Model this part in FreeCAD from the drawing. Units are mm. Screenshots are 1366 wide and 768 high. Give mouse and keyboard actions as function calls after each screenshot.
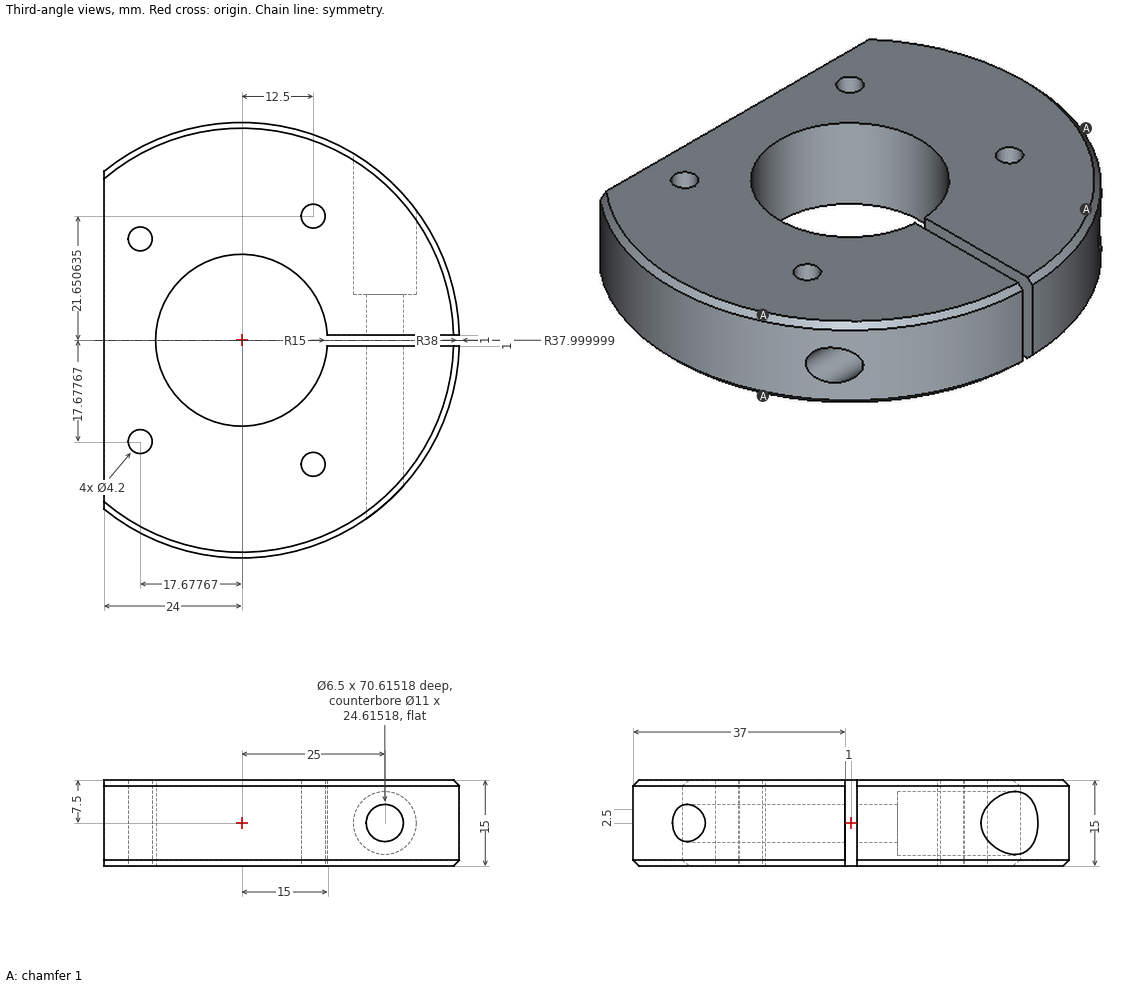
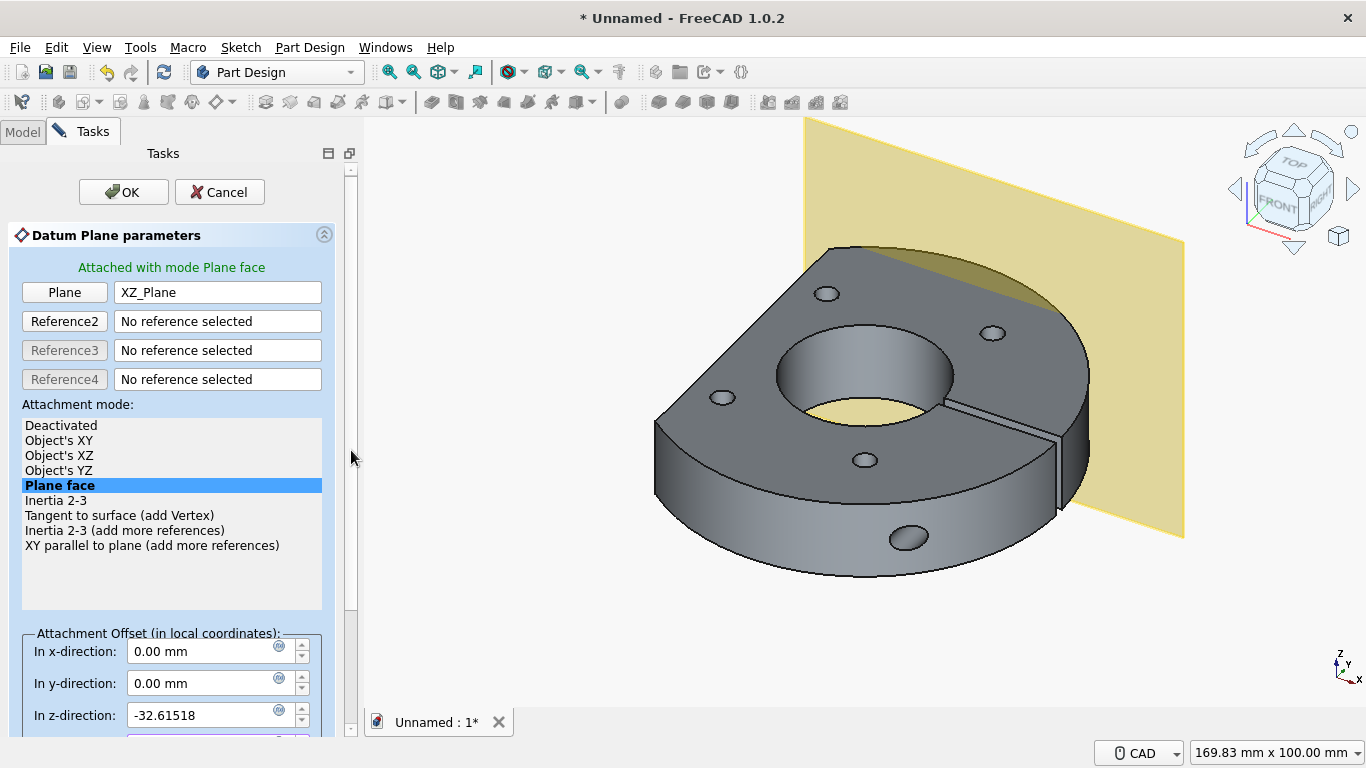
click(124, 192)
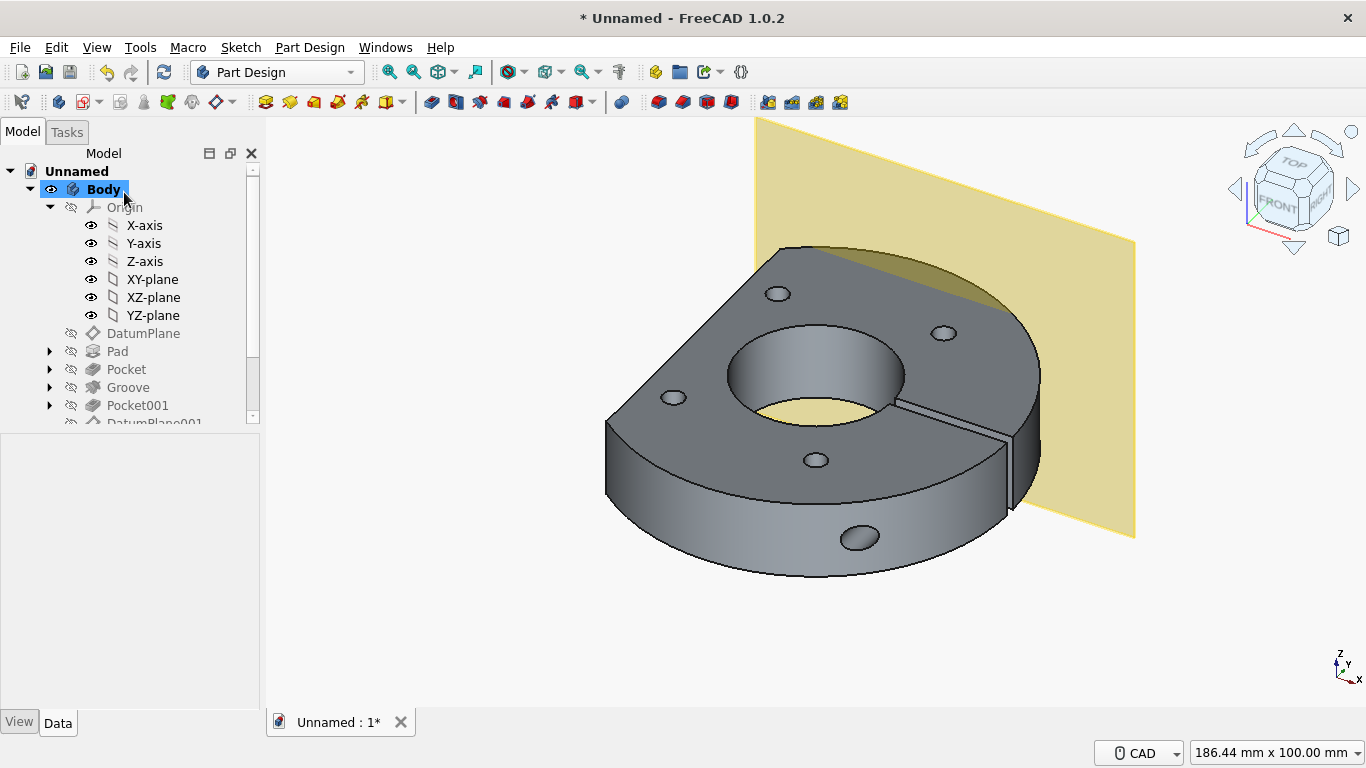
scroll(100, 293, down, 3)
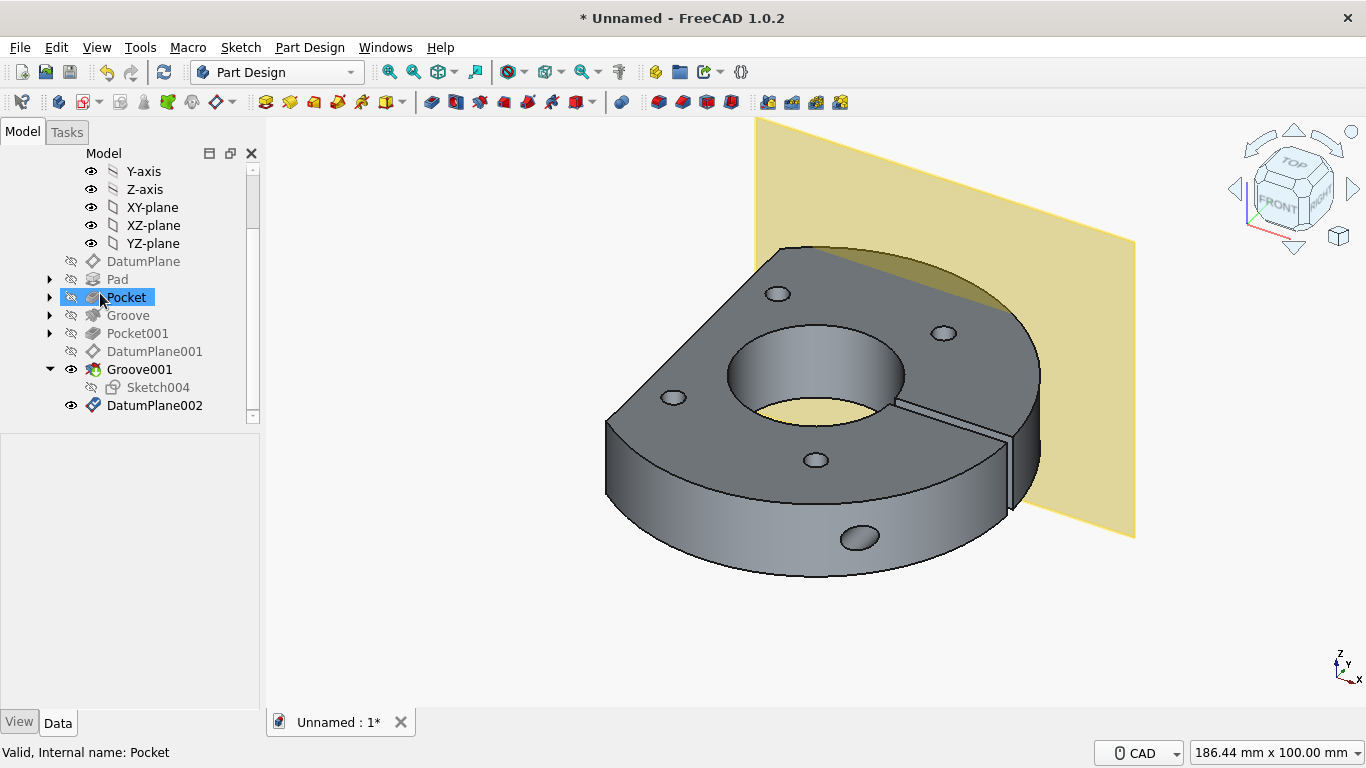
click(116, 405)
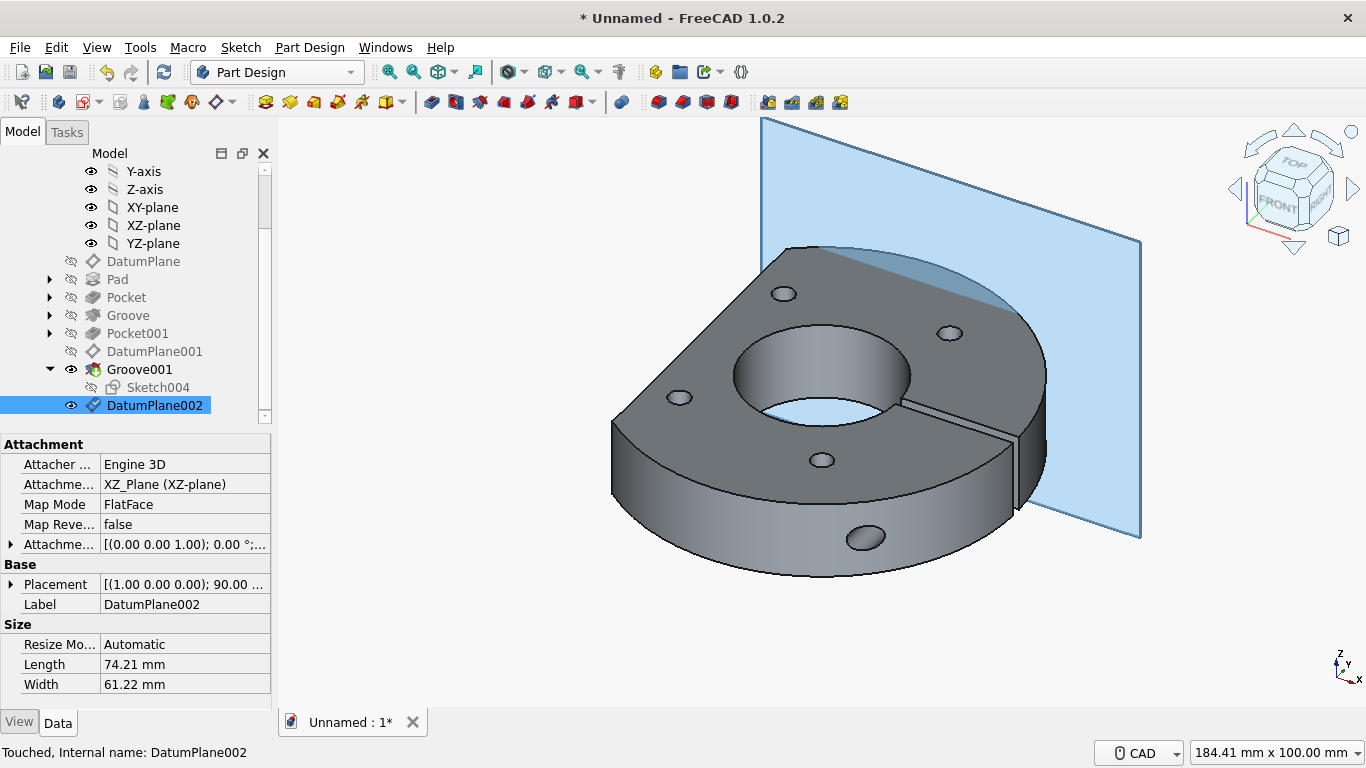
click(84, 102)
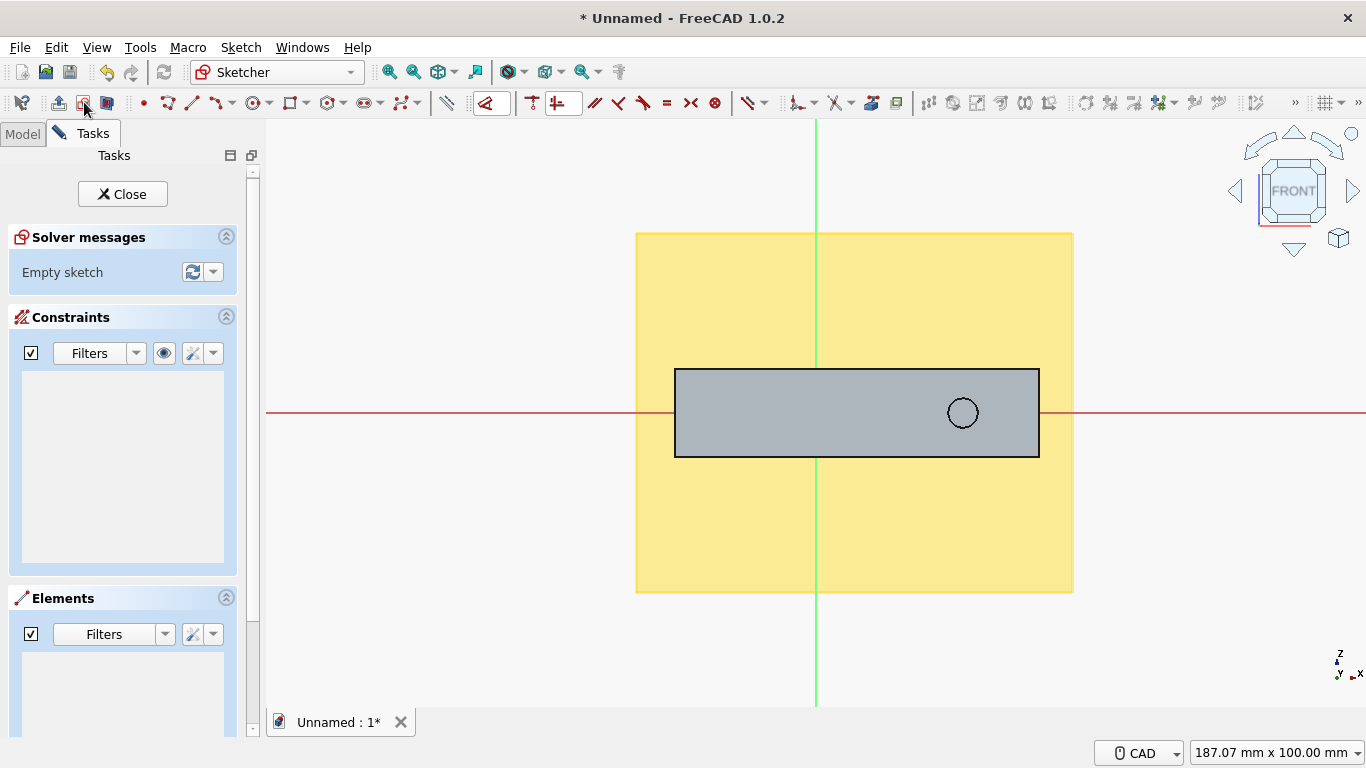
click(108, 104)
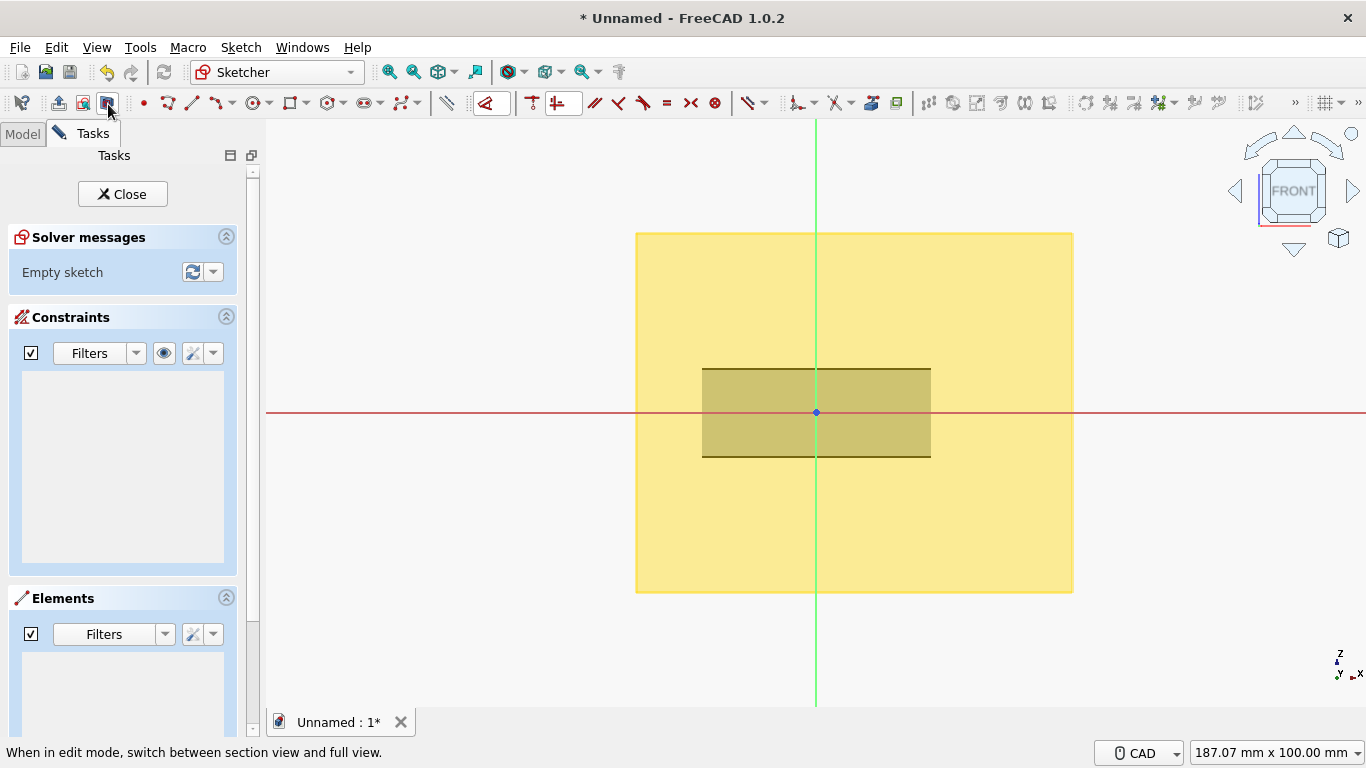
scroll(990, 413, up, 11)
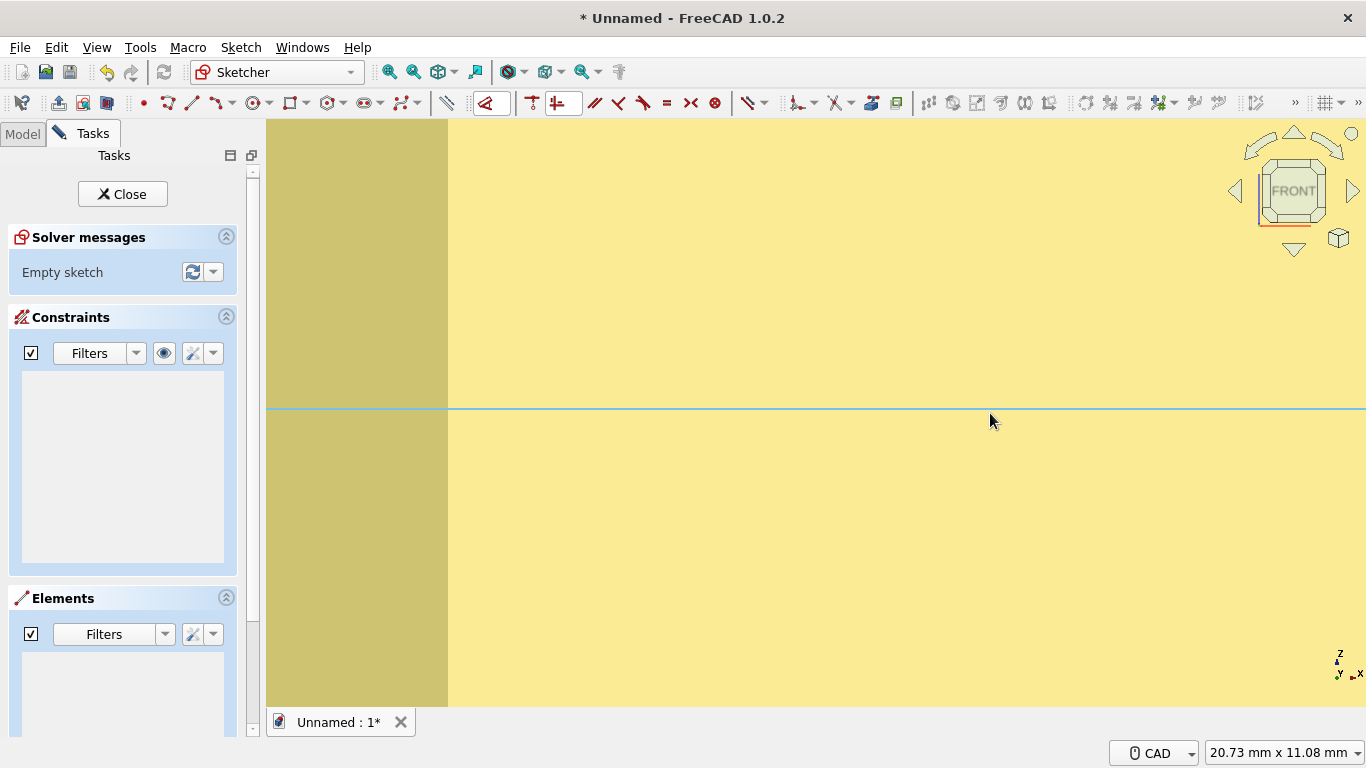
click(254, 104)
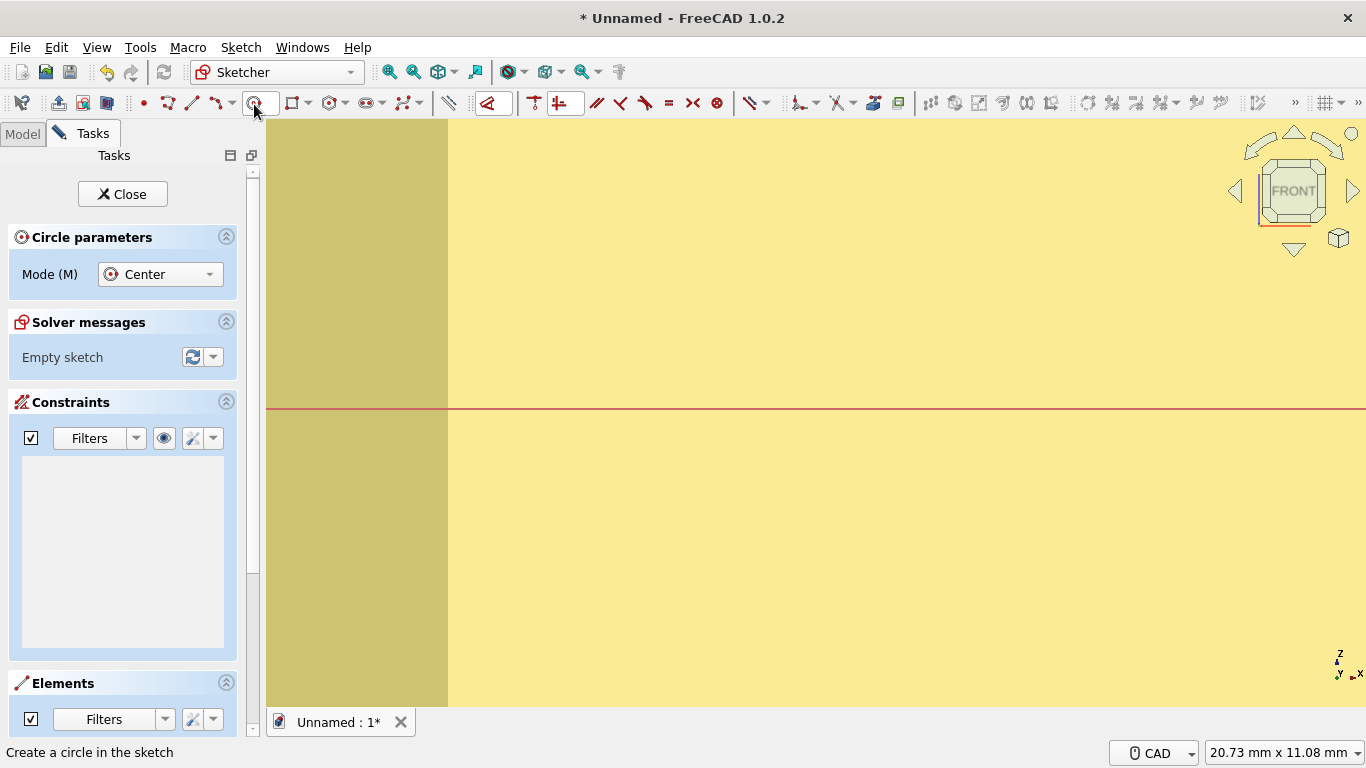
click(741, 409)
move(863, 287)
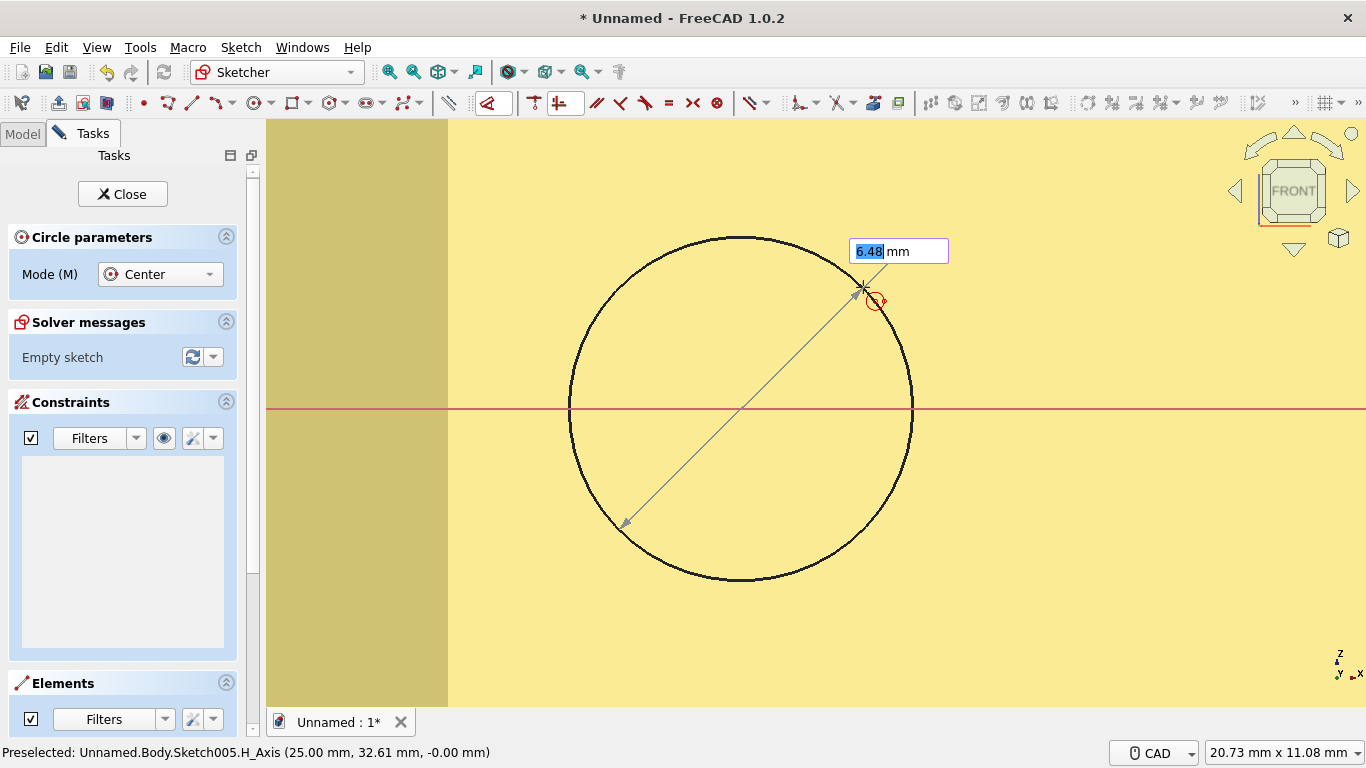
text(6.5)
key(Return)
key(Escape)